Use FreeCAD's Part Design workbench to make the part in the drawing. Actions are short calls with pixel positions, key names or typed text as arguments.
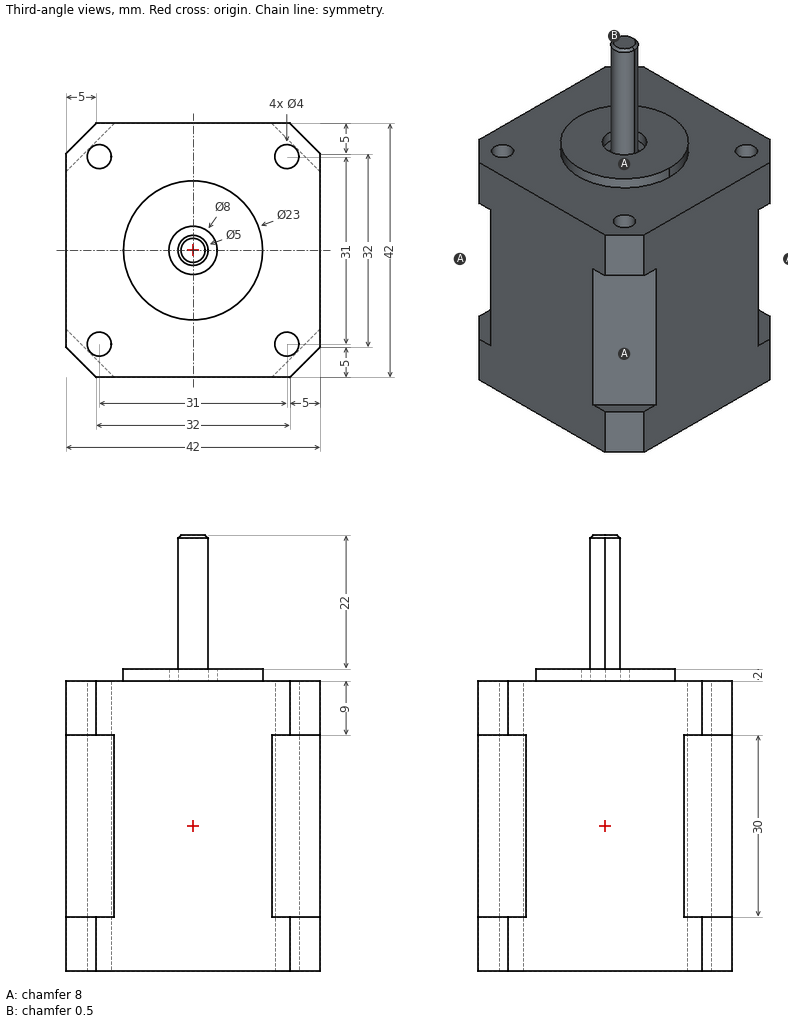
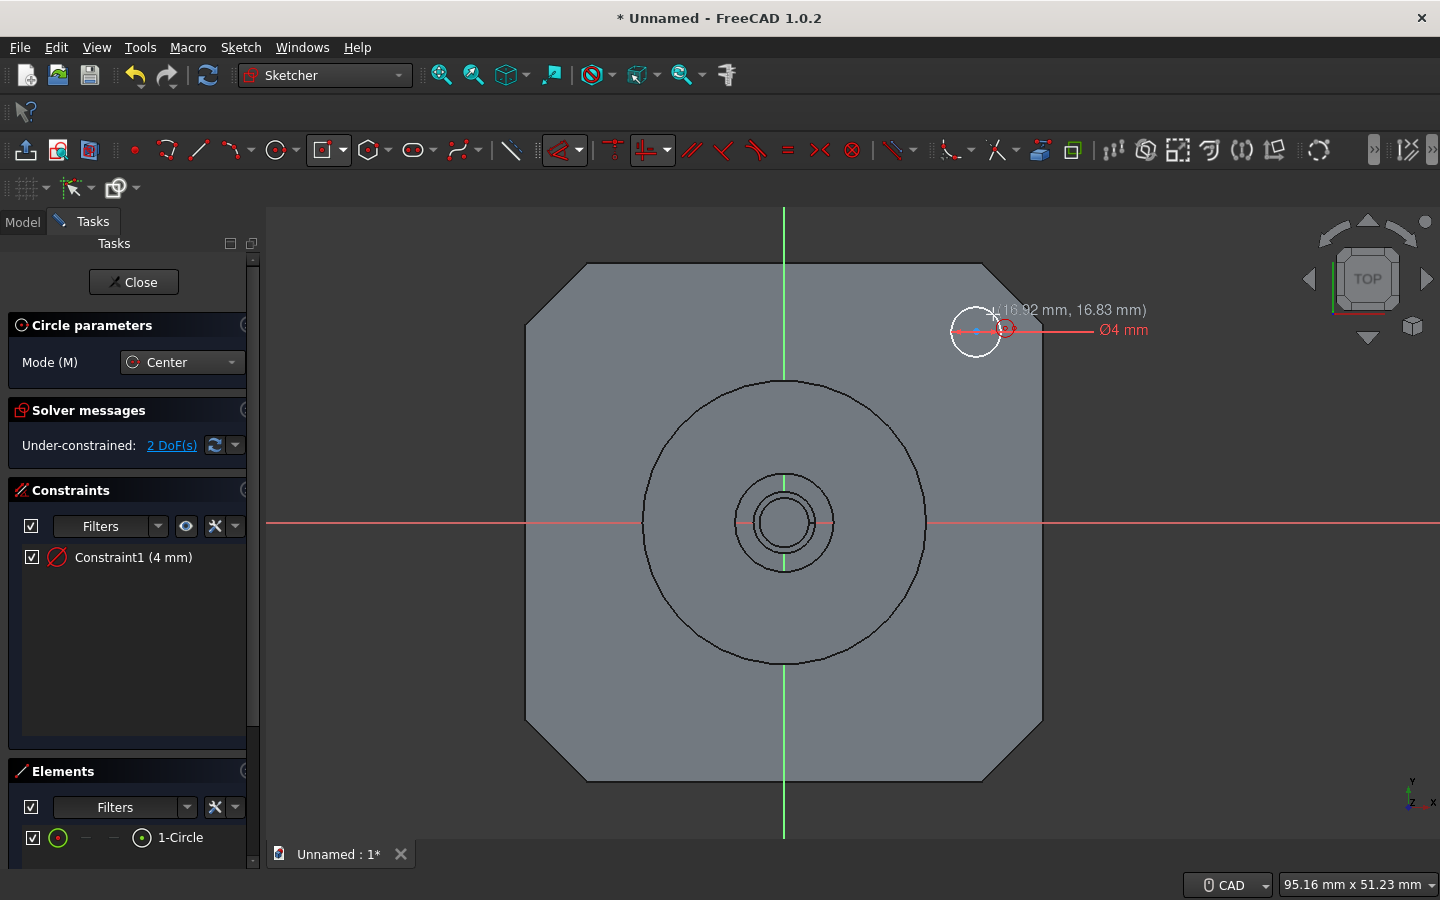
click(976, 714)
move(993, 696)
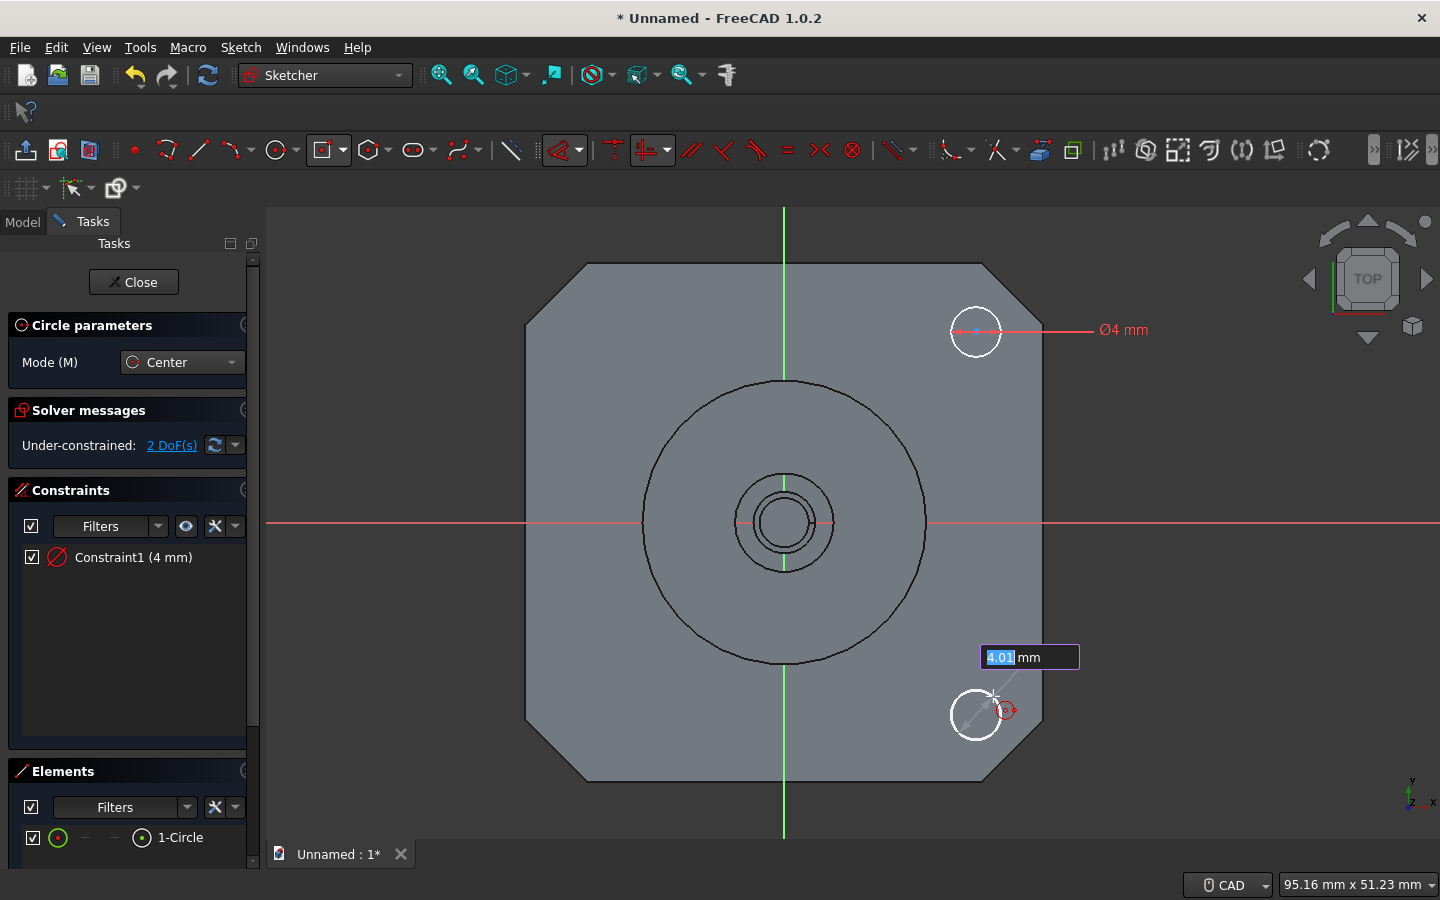
text(4)
key(Return)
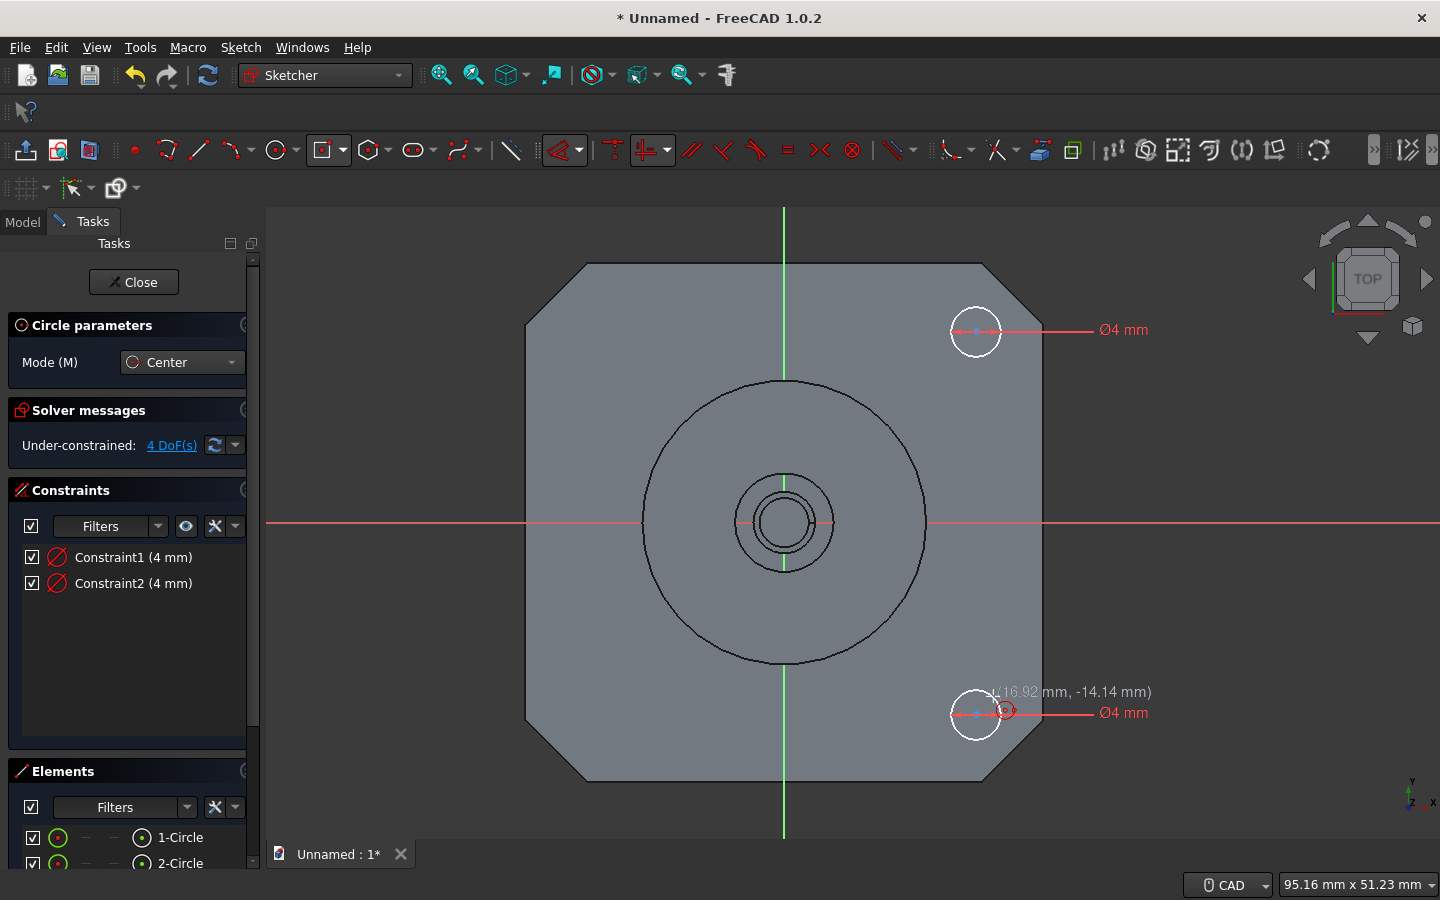
click(593, 714)
move(611, 696)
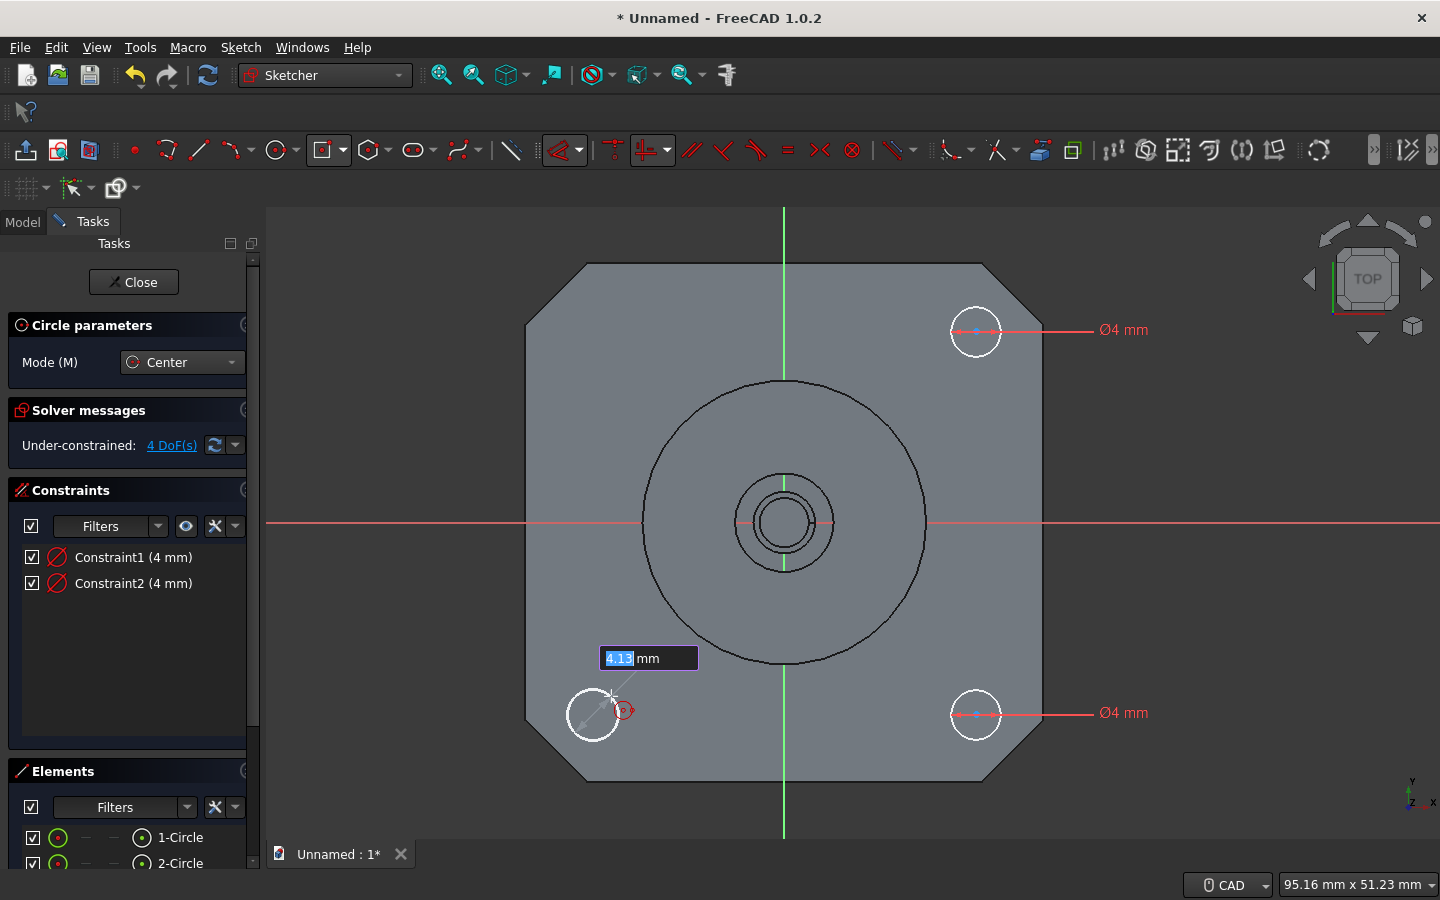
text(4)
key(Return)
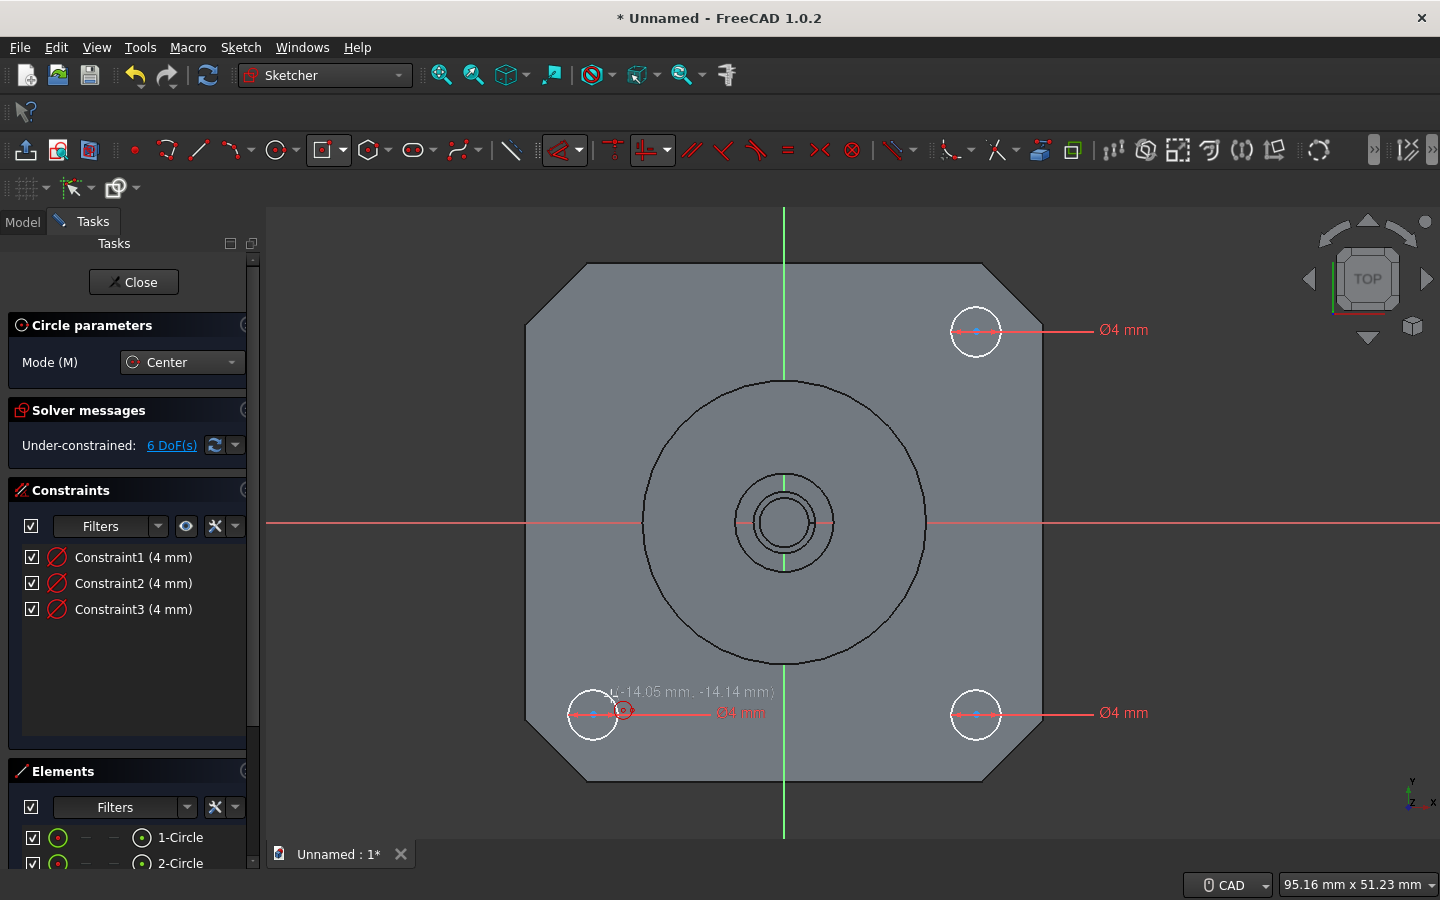
click(593, 331)
move(611, 314)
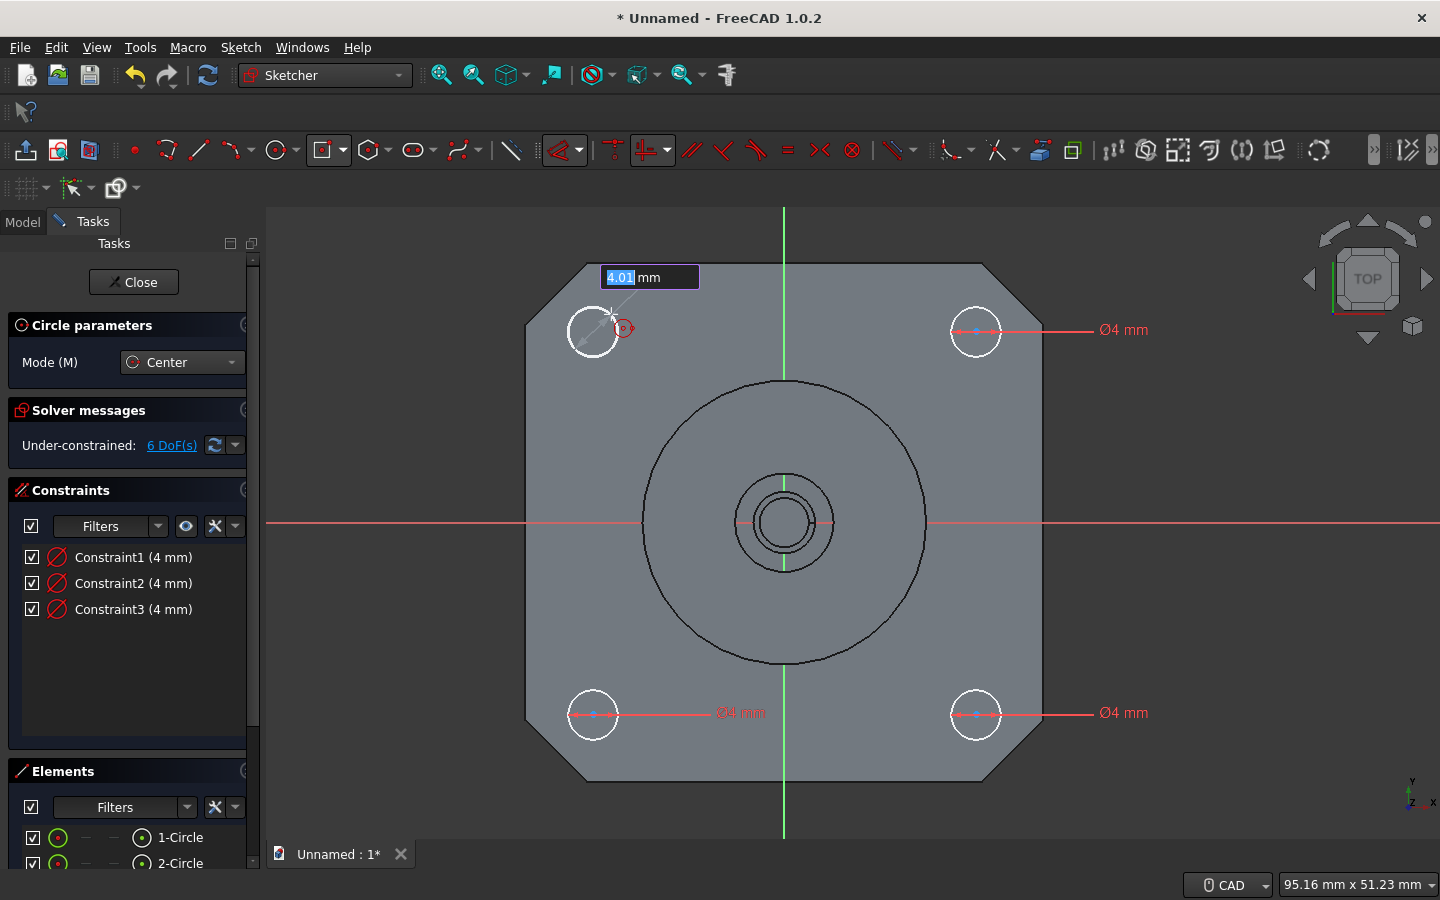
text(4)
key(Return)
key(Escape)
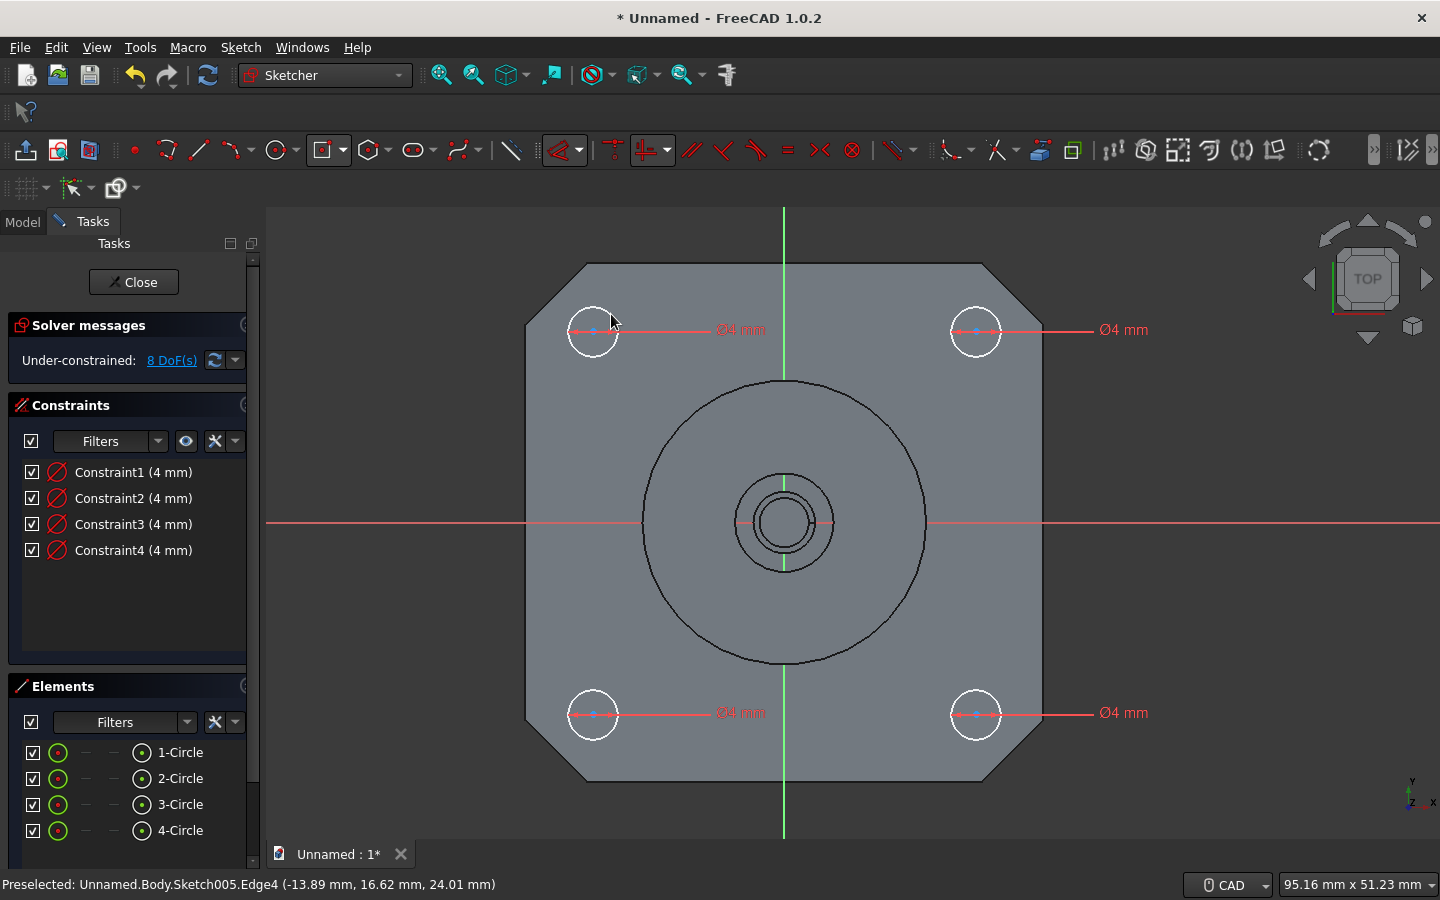
click(976, 332)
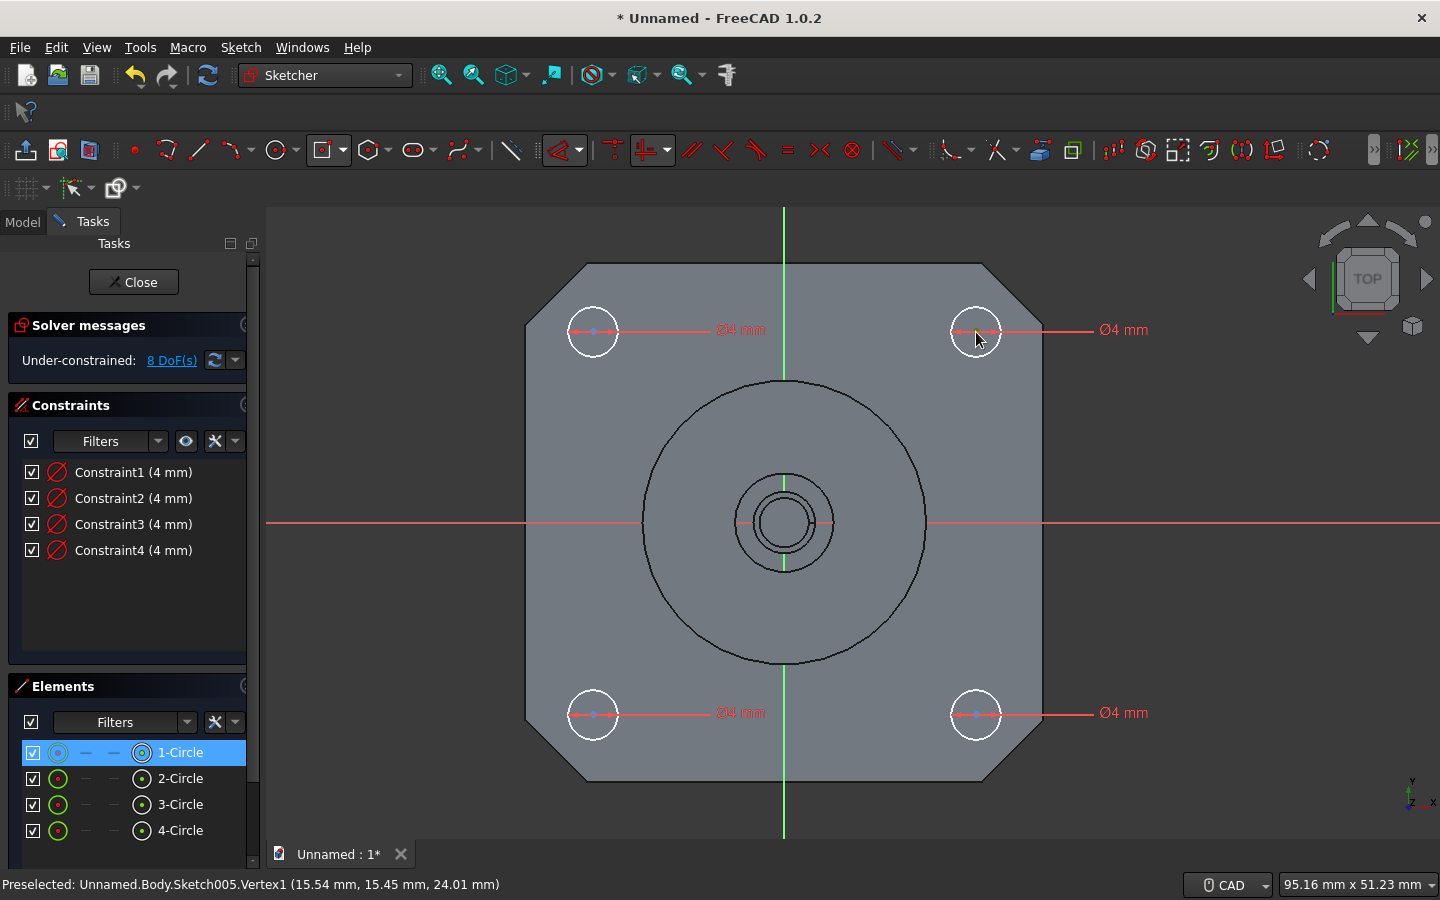
click(976, 715)